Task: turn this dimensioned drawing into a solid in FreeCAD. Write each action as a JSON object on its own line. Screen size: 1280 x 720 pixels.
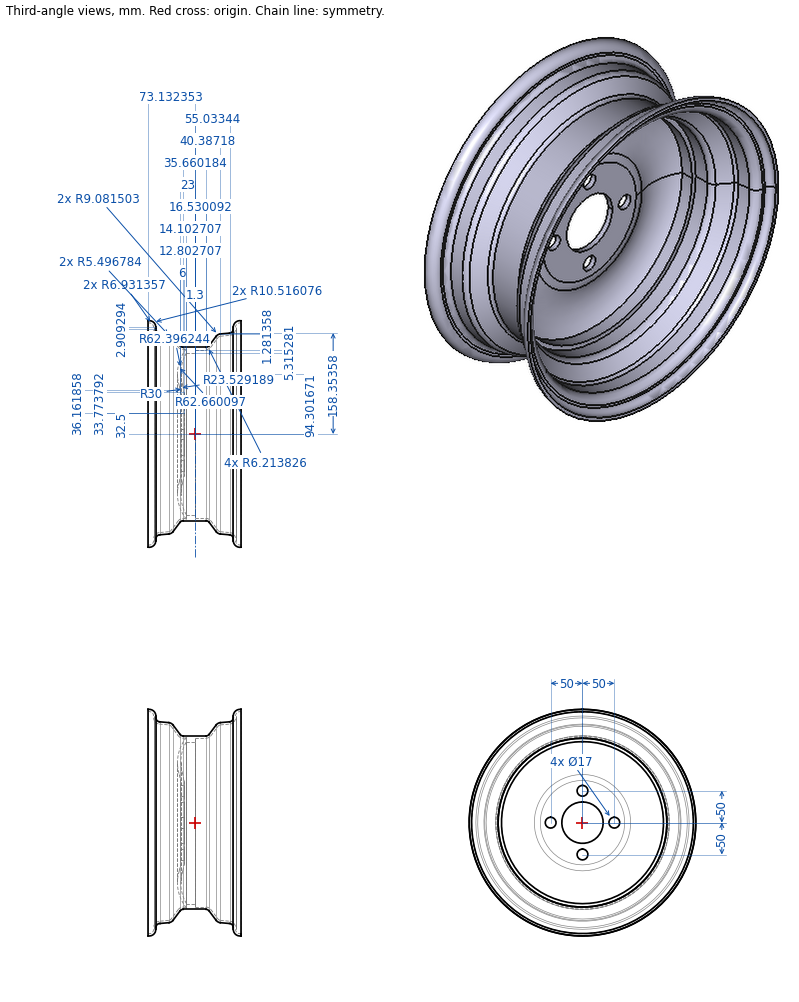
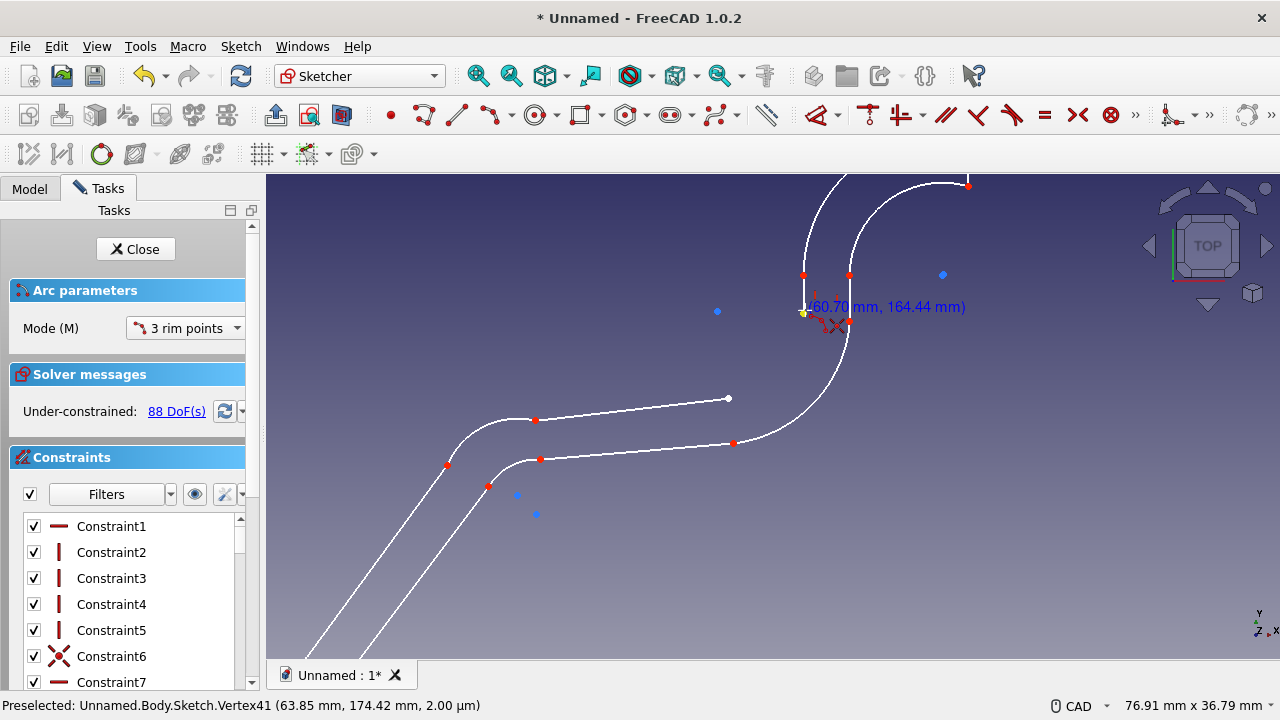
{"action": "left_click", "coordinate": [804, 313]}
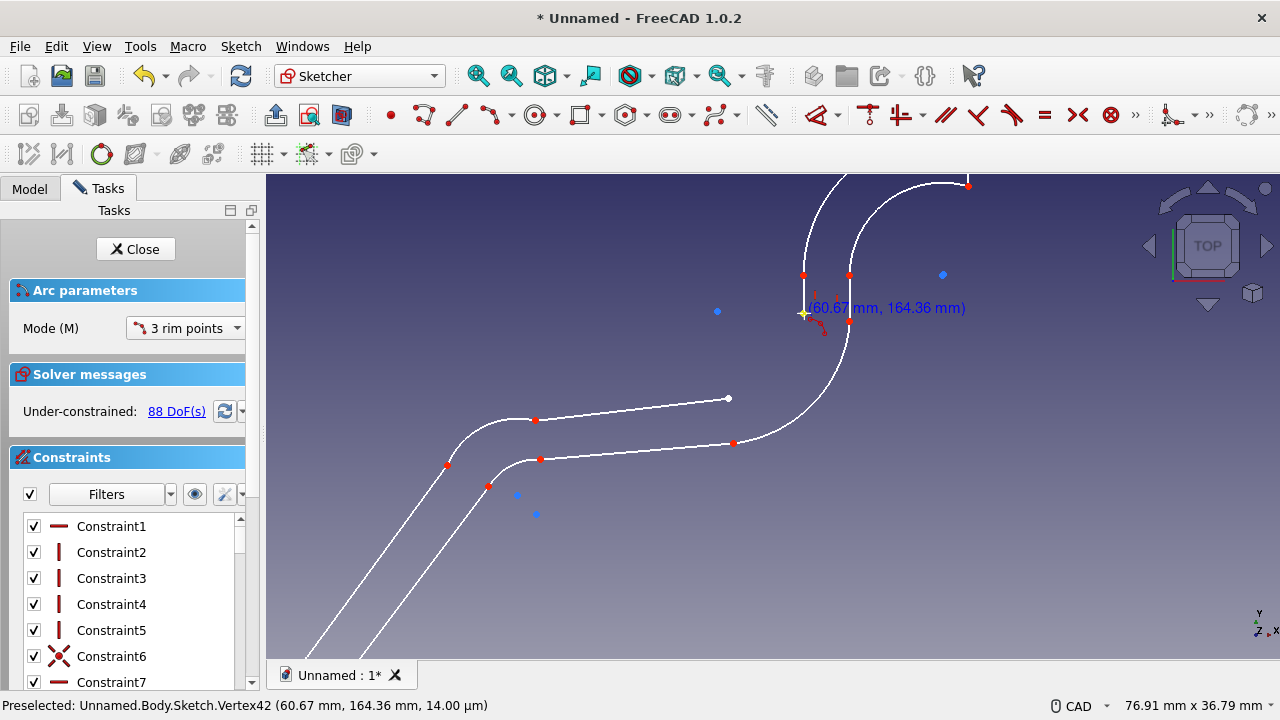
{"action": "scroll", "coordinate": [814, 277], "scroll_direction": "down", "scroll_amount": 10}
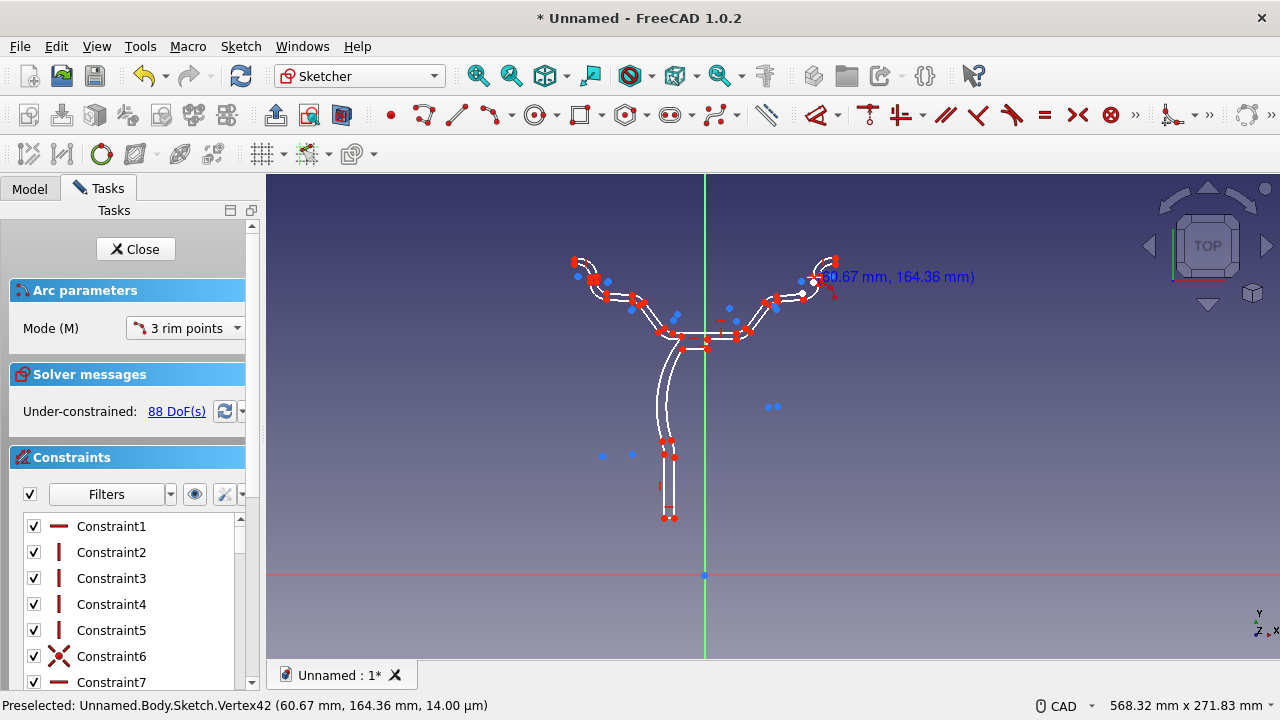
{"action": "scroll", "coordinate": [803, 293], "scroll_direction": "up", "scroll_amount": 5}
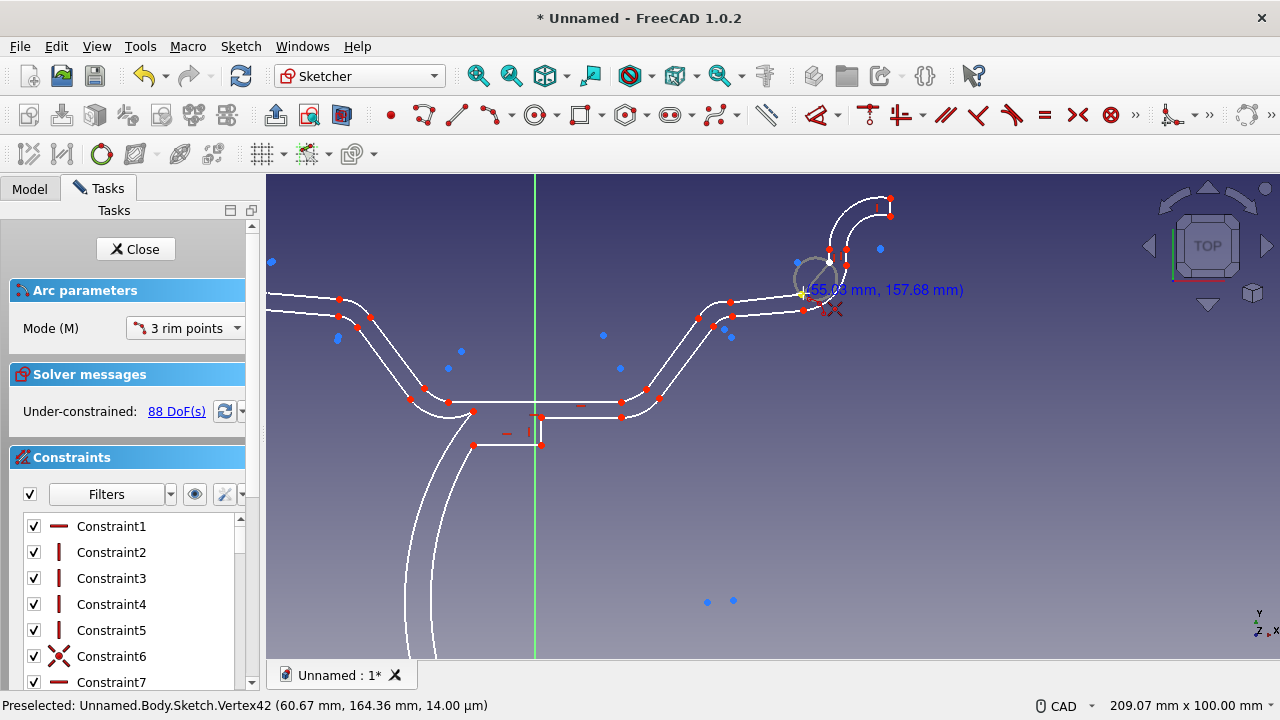
{"action": "left_click", "coordinate": [802, 294]}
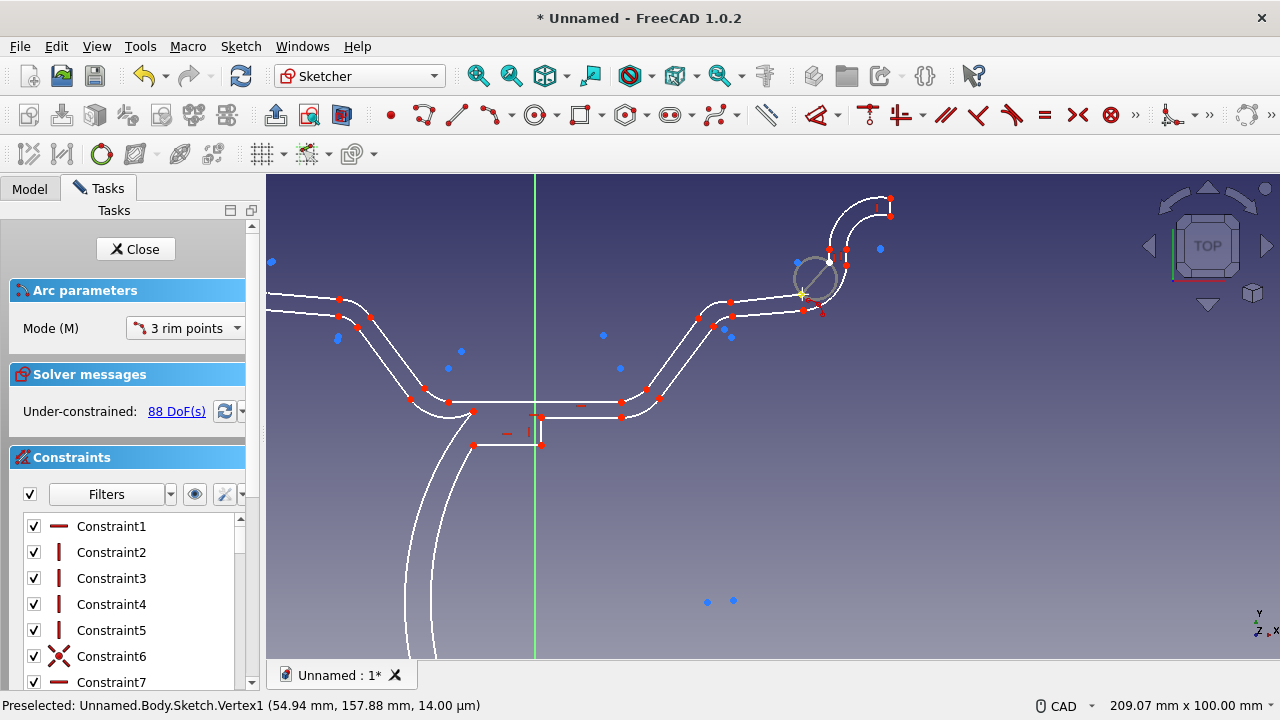
{"action": "scroll", "coordinate": [822, 282], "scroll_direction": "up", "scroll_amount": 4}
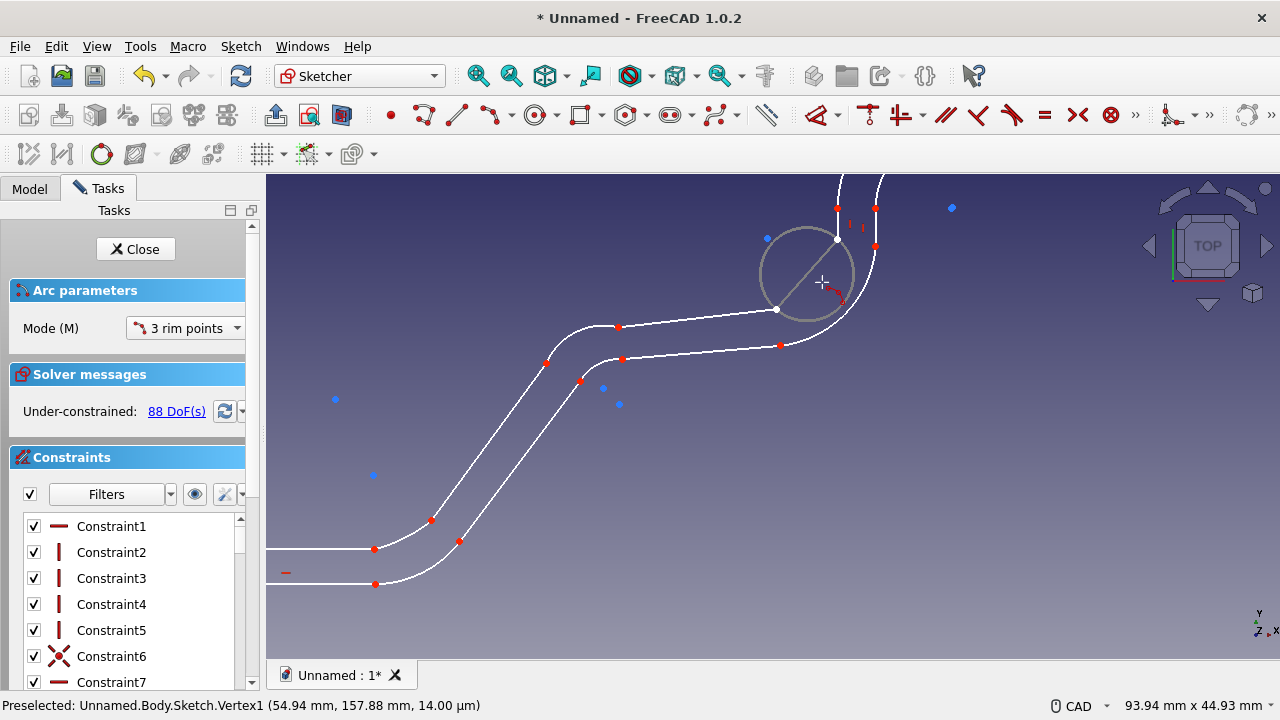
{"action": "left_click", "coordinate": [821, 283]}
{"action": "key", "text": "Escape"}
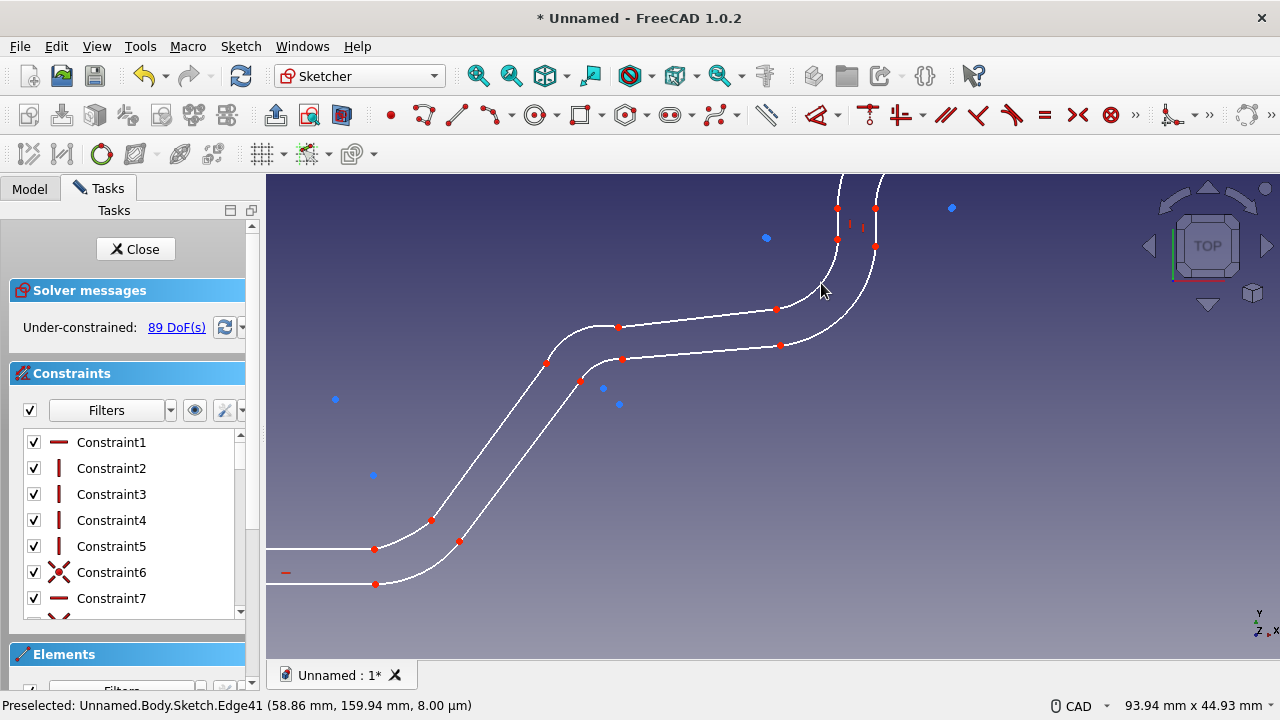
{"action": "left_click", "coordinate": [729, 315]}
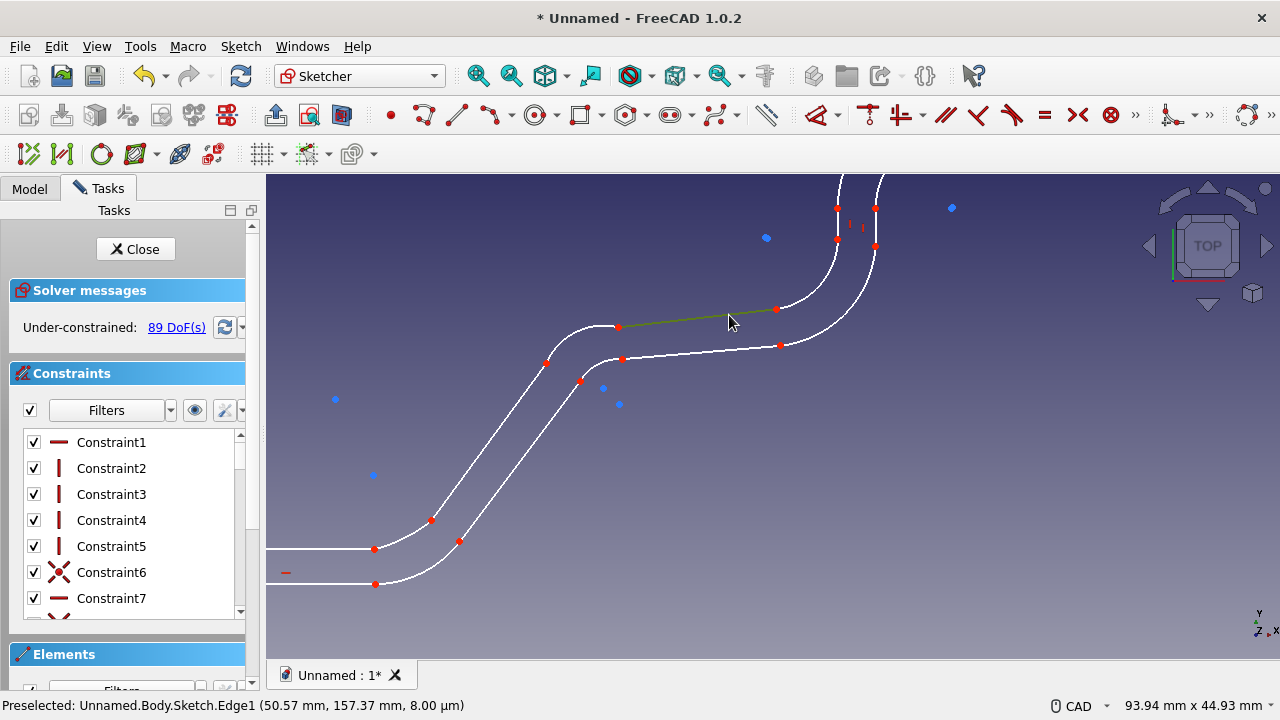
{"action": "left_click", "coordinate": [592, 327]}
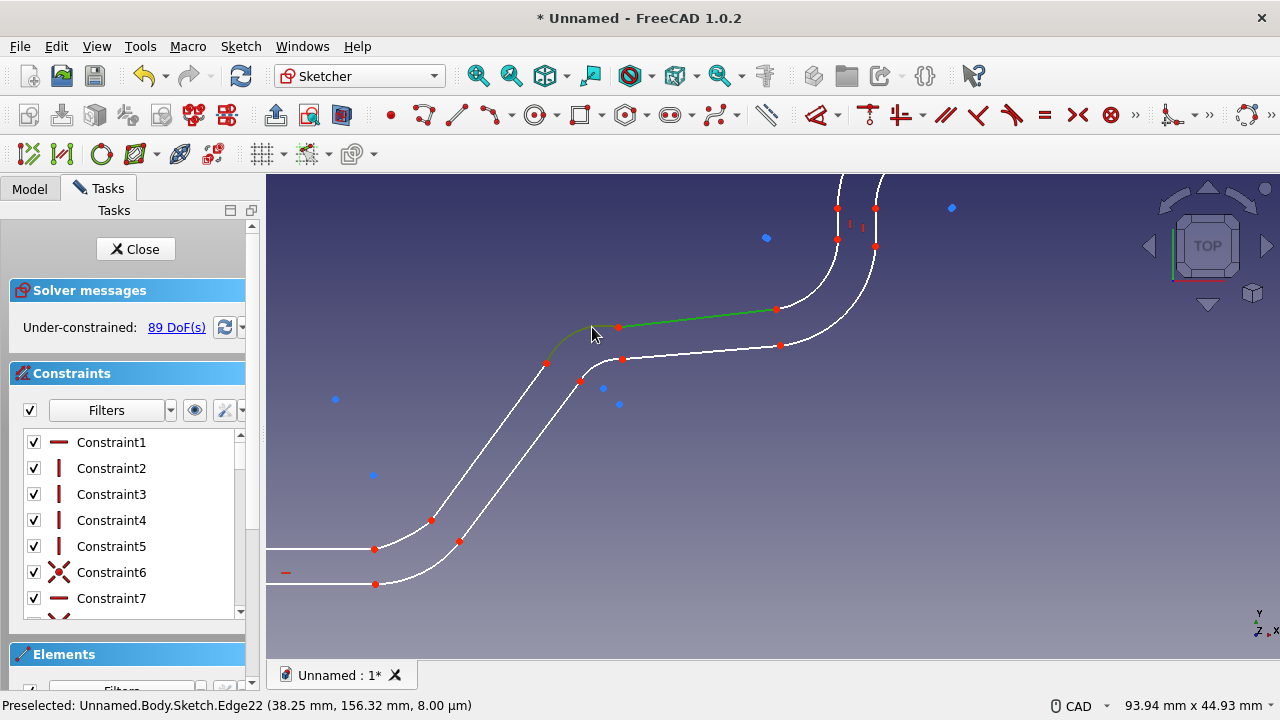
{"action": "key", "text": "t"}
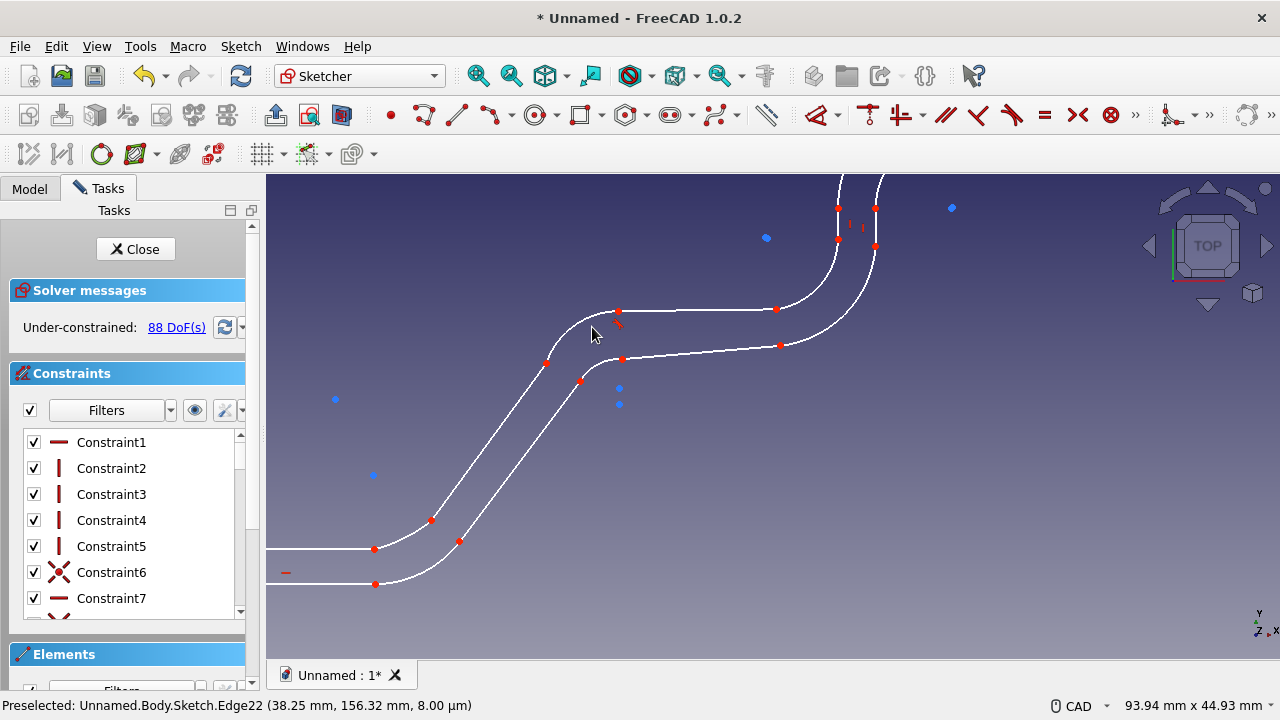
{"action": "scroll", "coordinate": [808, 290], "scroll_direction": "down", "scroll_amount": 9}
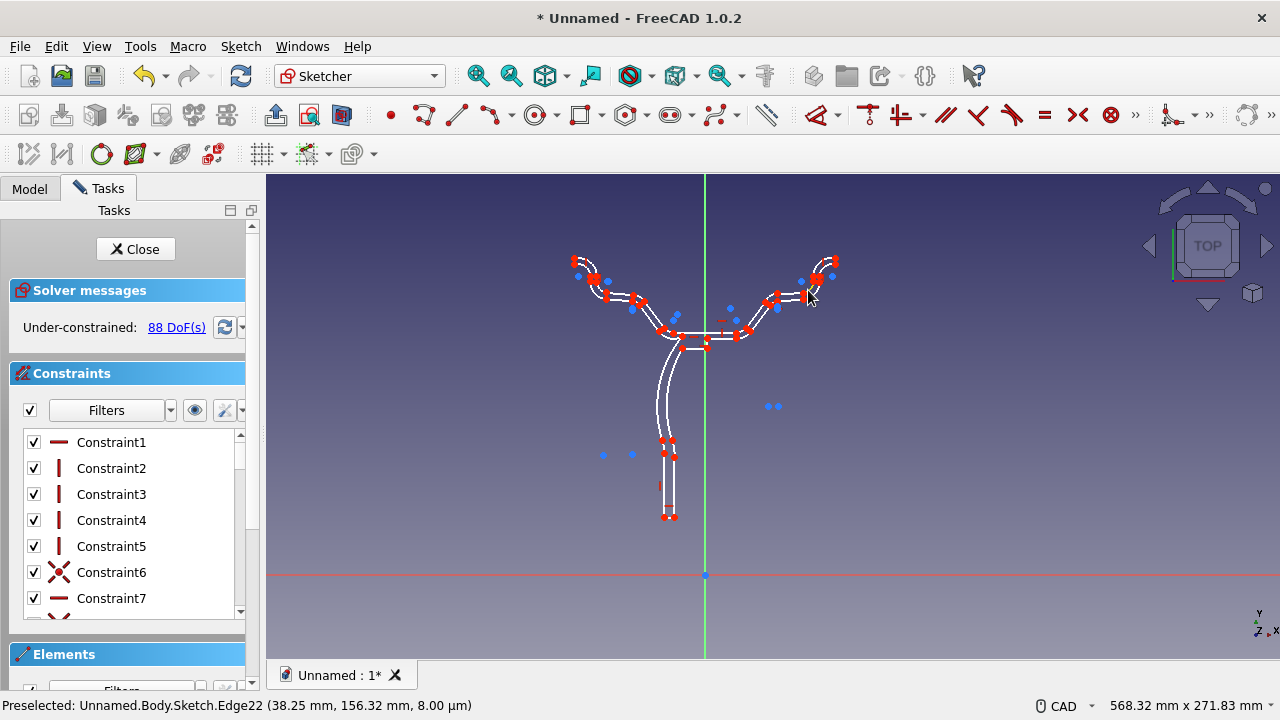
{"action": "scroll", "coordinate": [795, 293], "scroll_direction": "up", "scroll_amount": 4}